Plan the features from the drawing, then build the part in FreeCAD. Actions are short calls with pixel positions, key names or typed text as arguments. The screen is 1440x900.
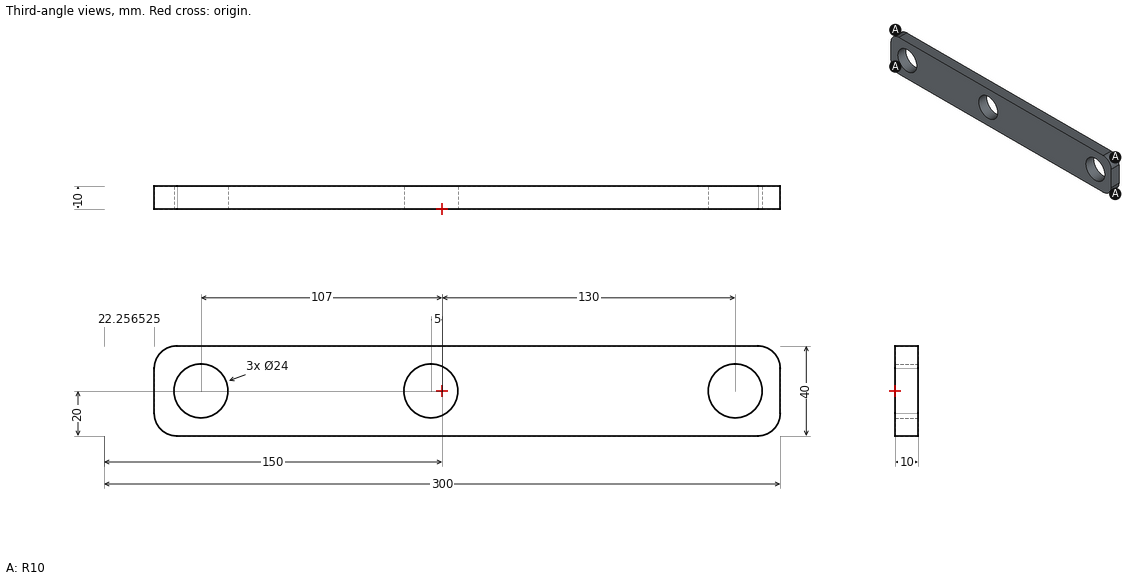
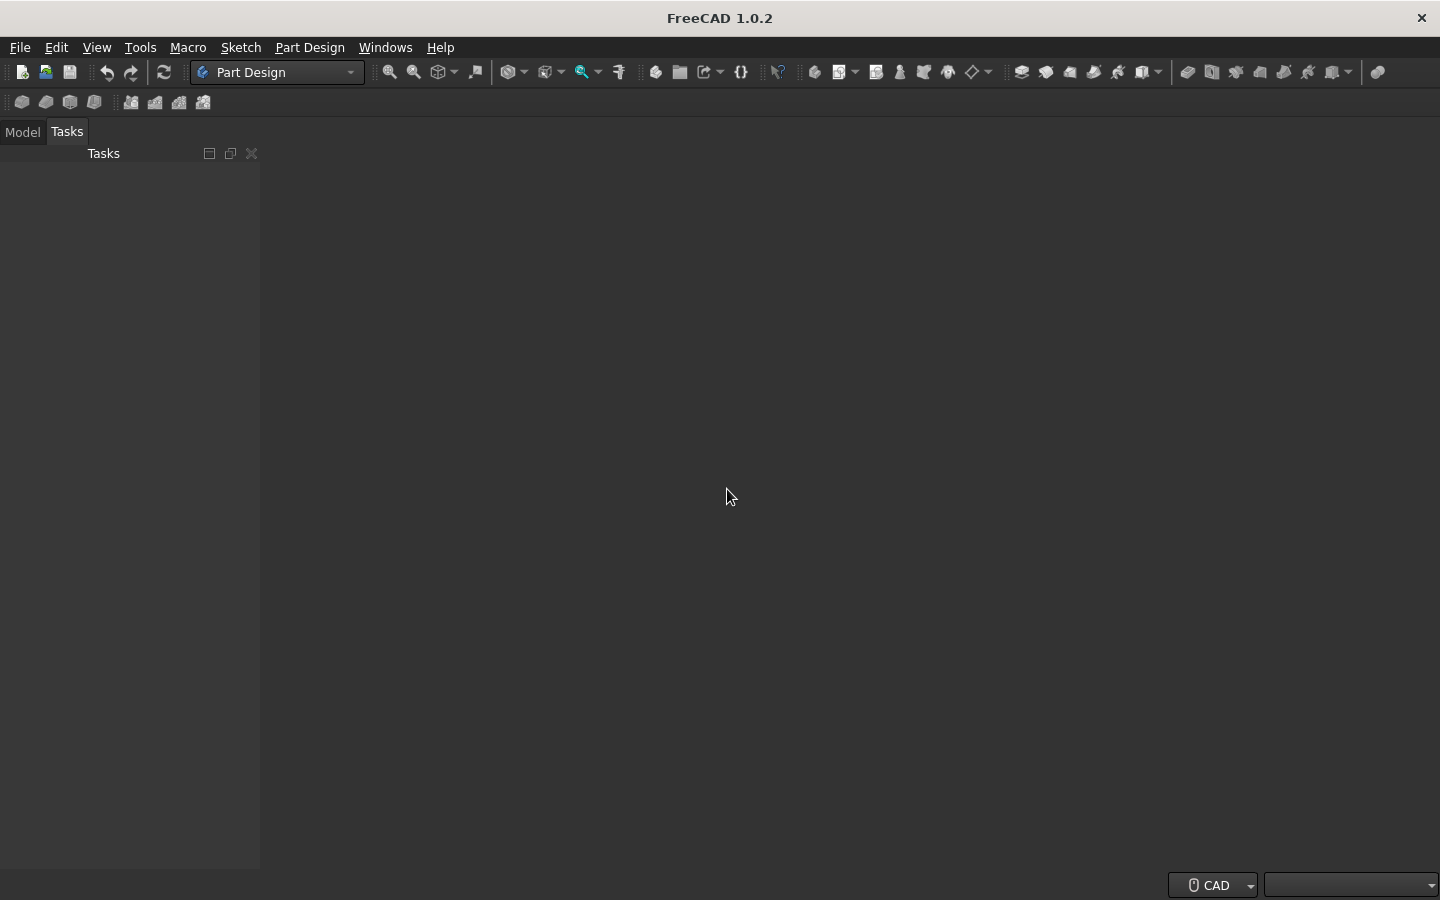
click(22, 72)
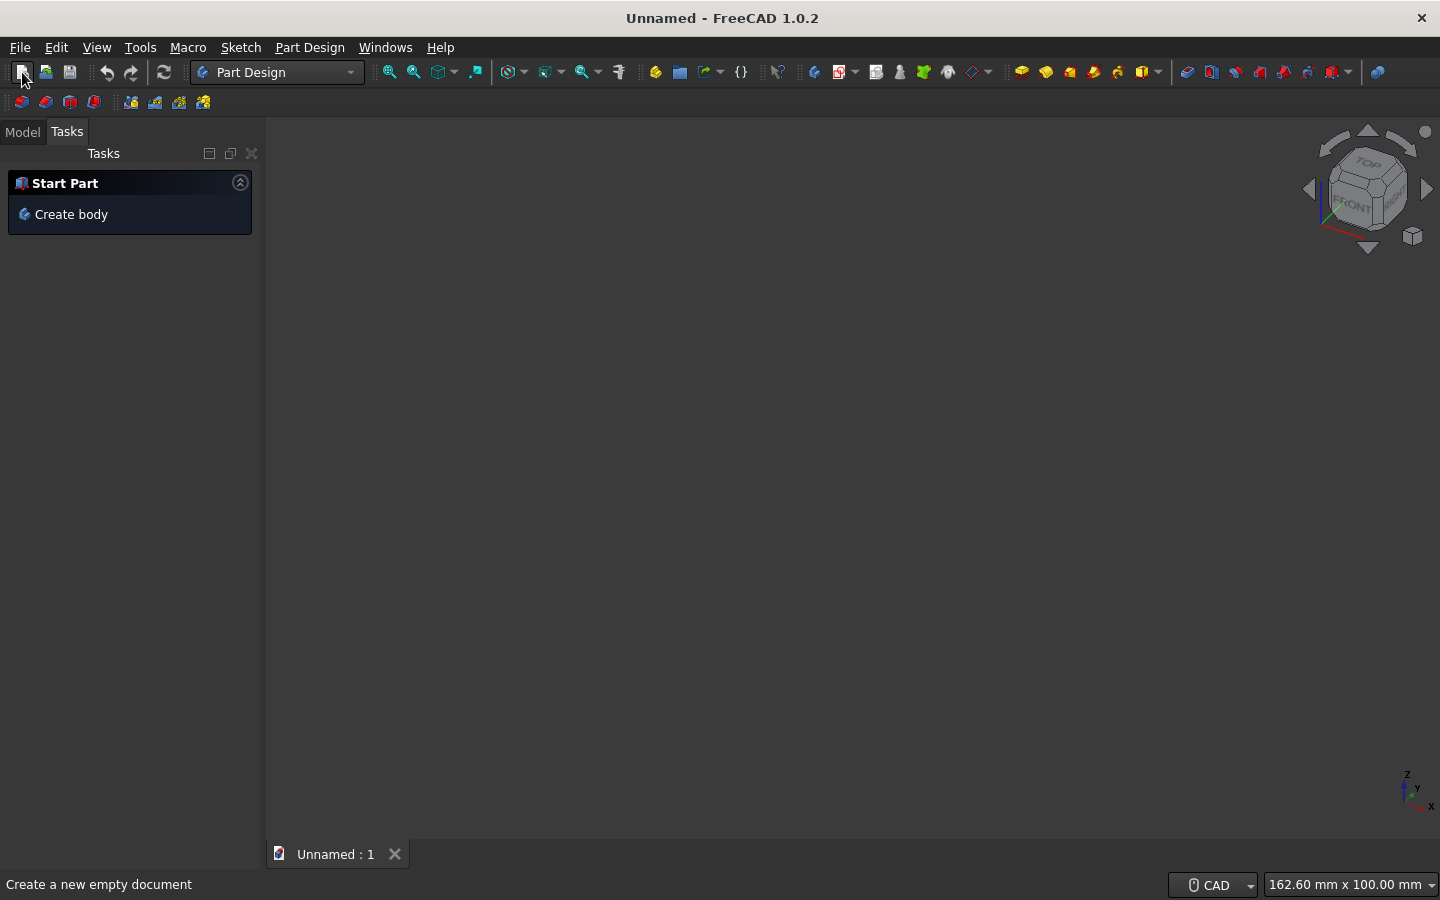
click(840, 72)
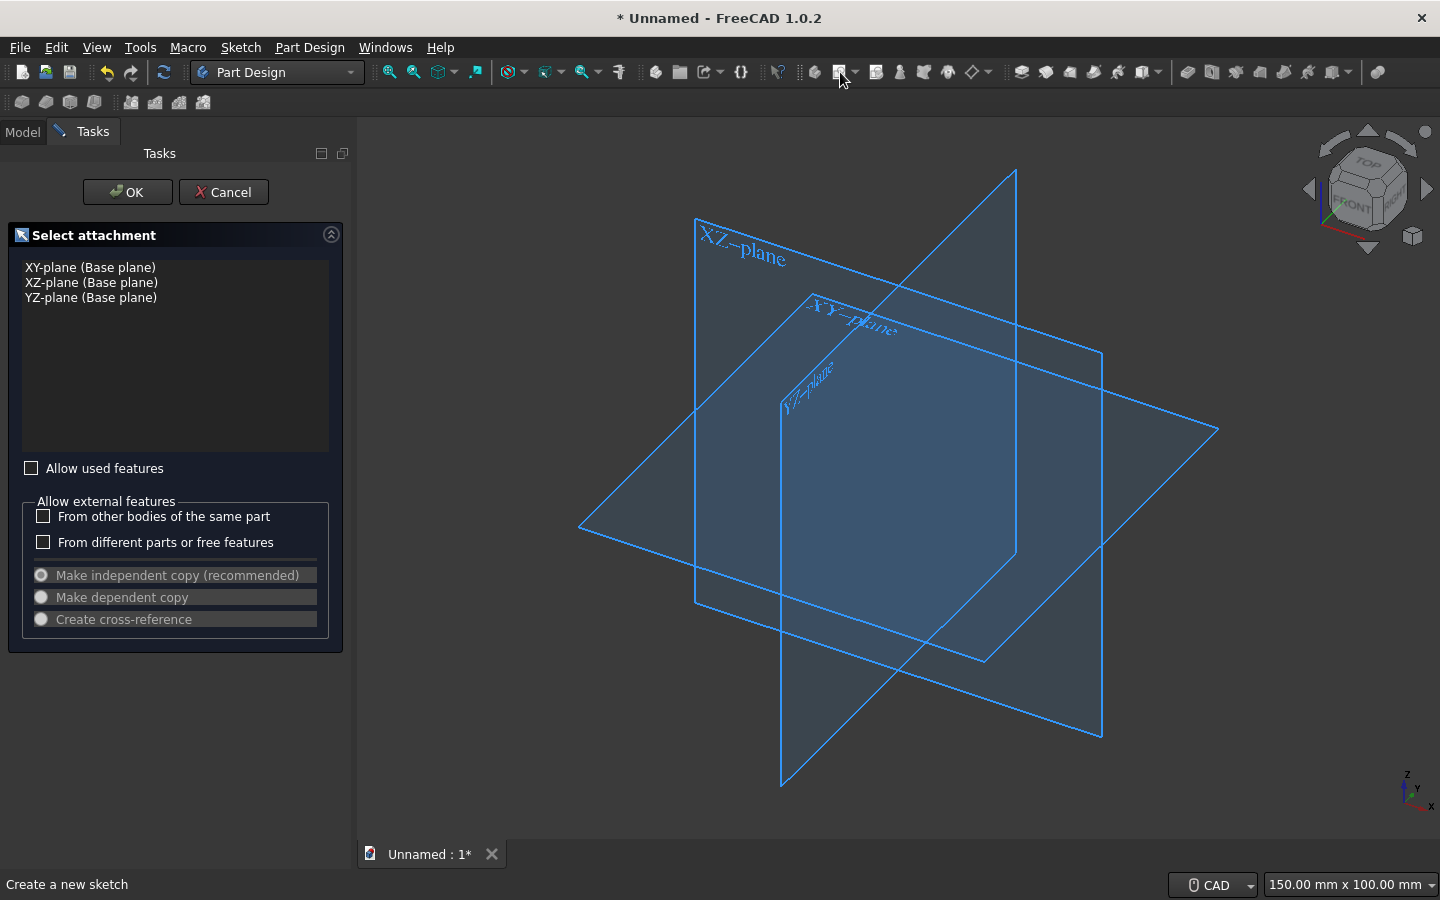
click(82, 282)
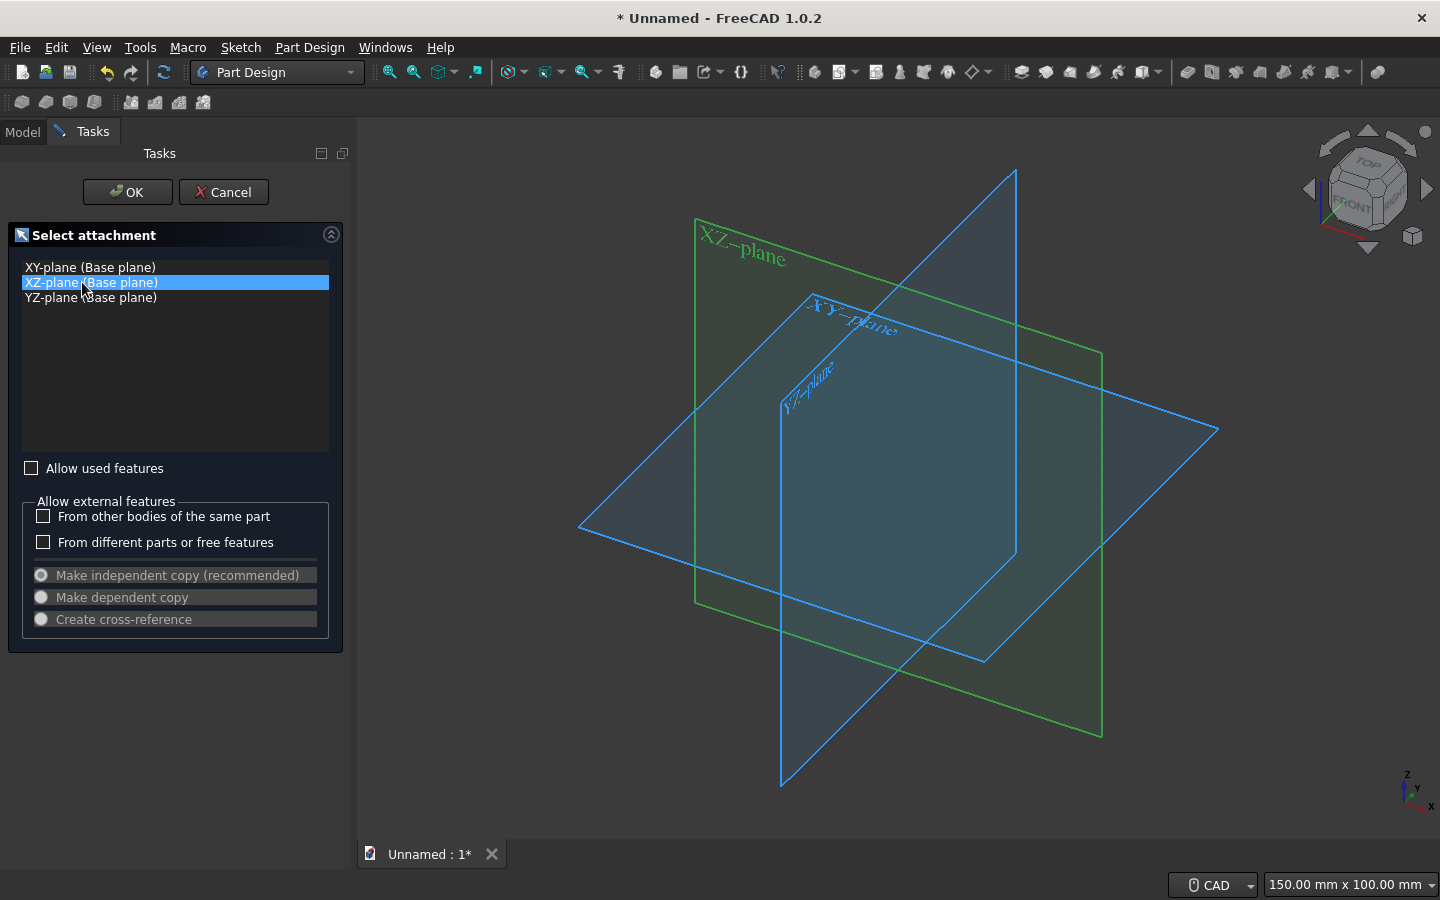
click(128, 192)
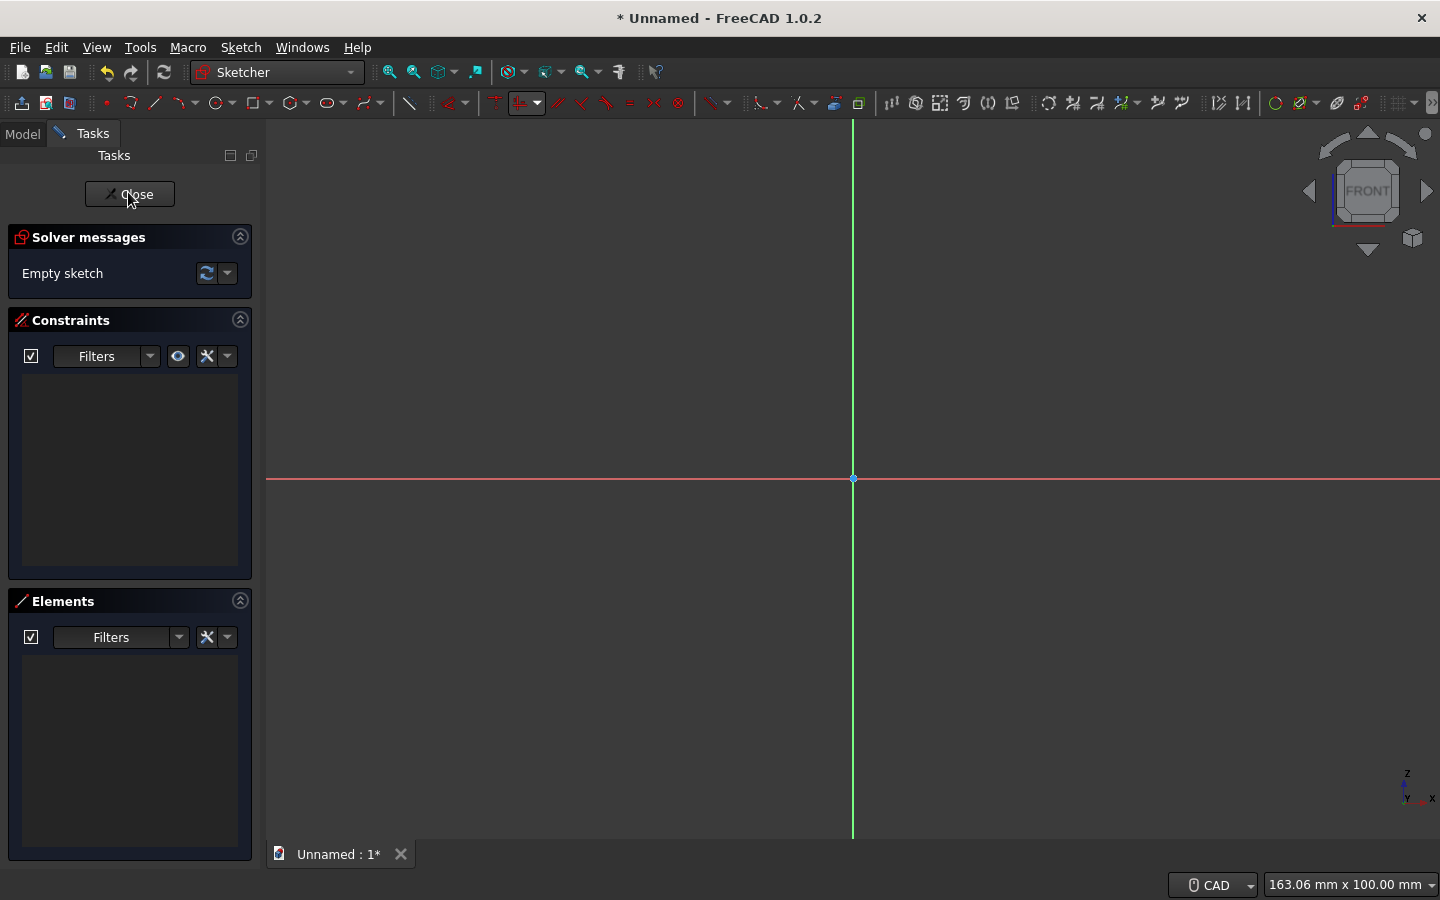
scroll(755, 479, down, 6)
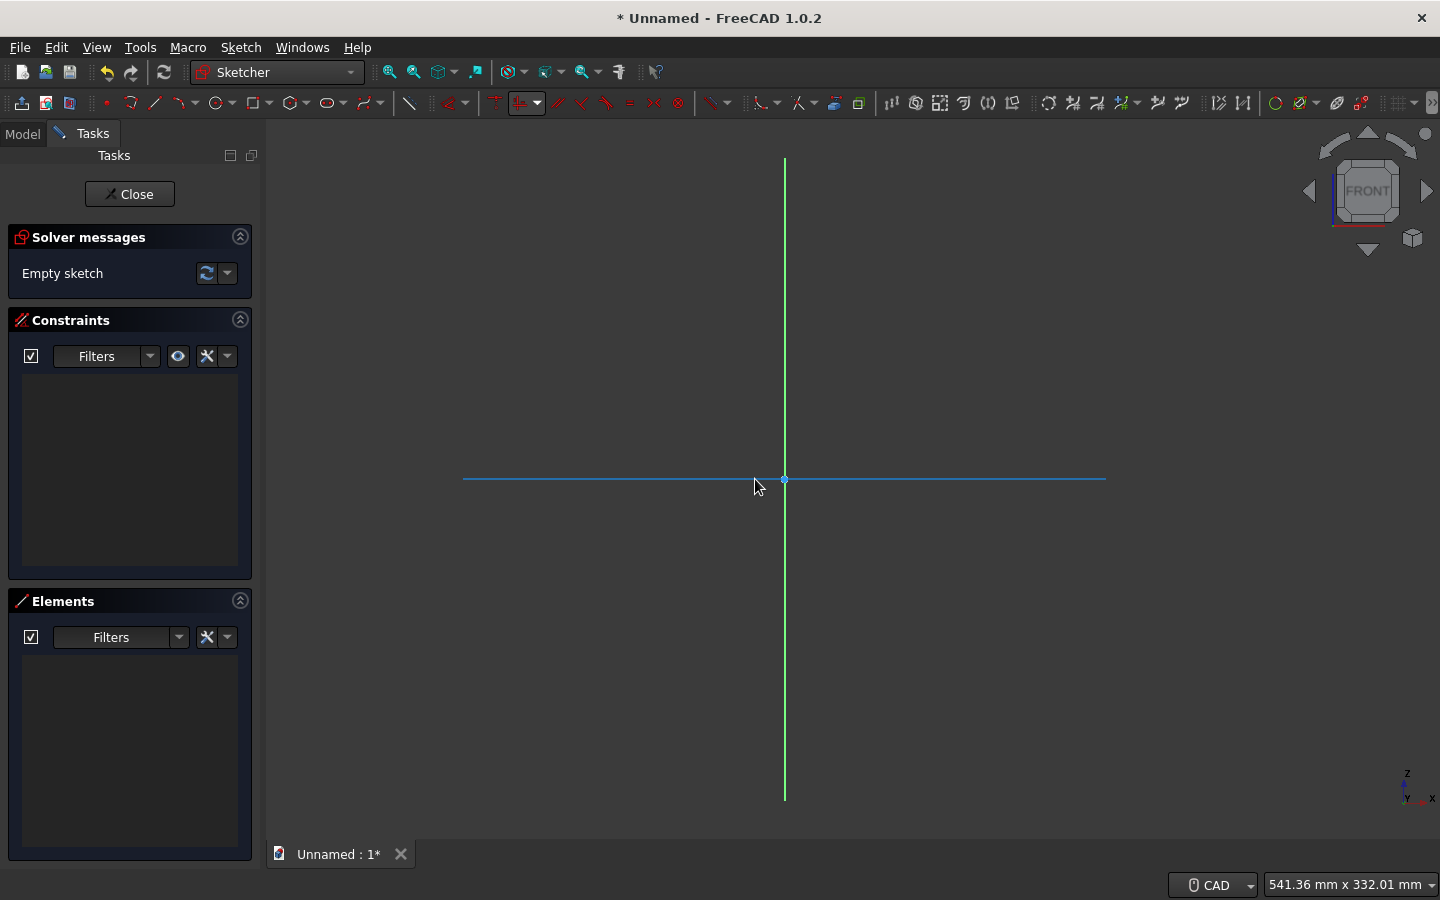
key(g)
key(v)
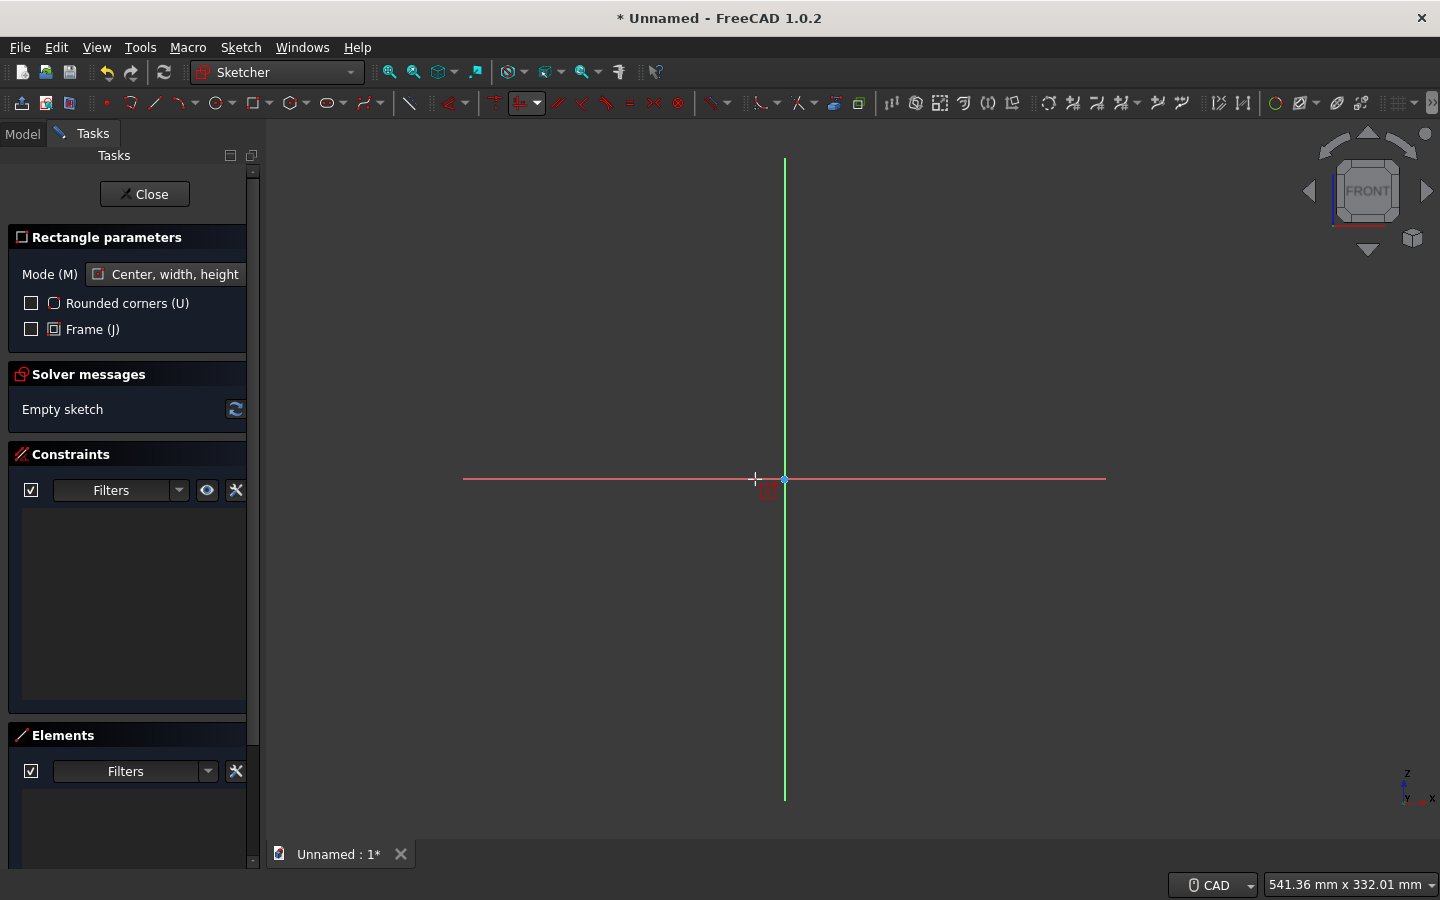
click(785, 479)
click(1110, 436)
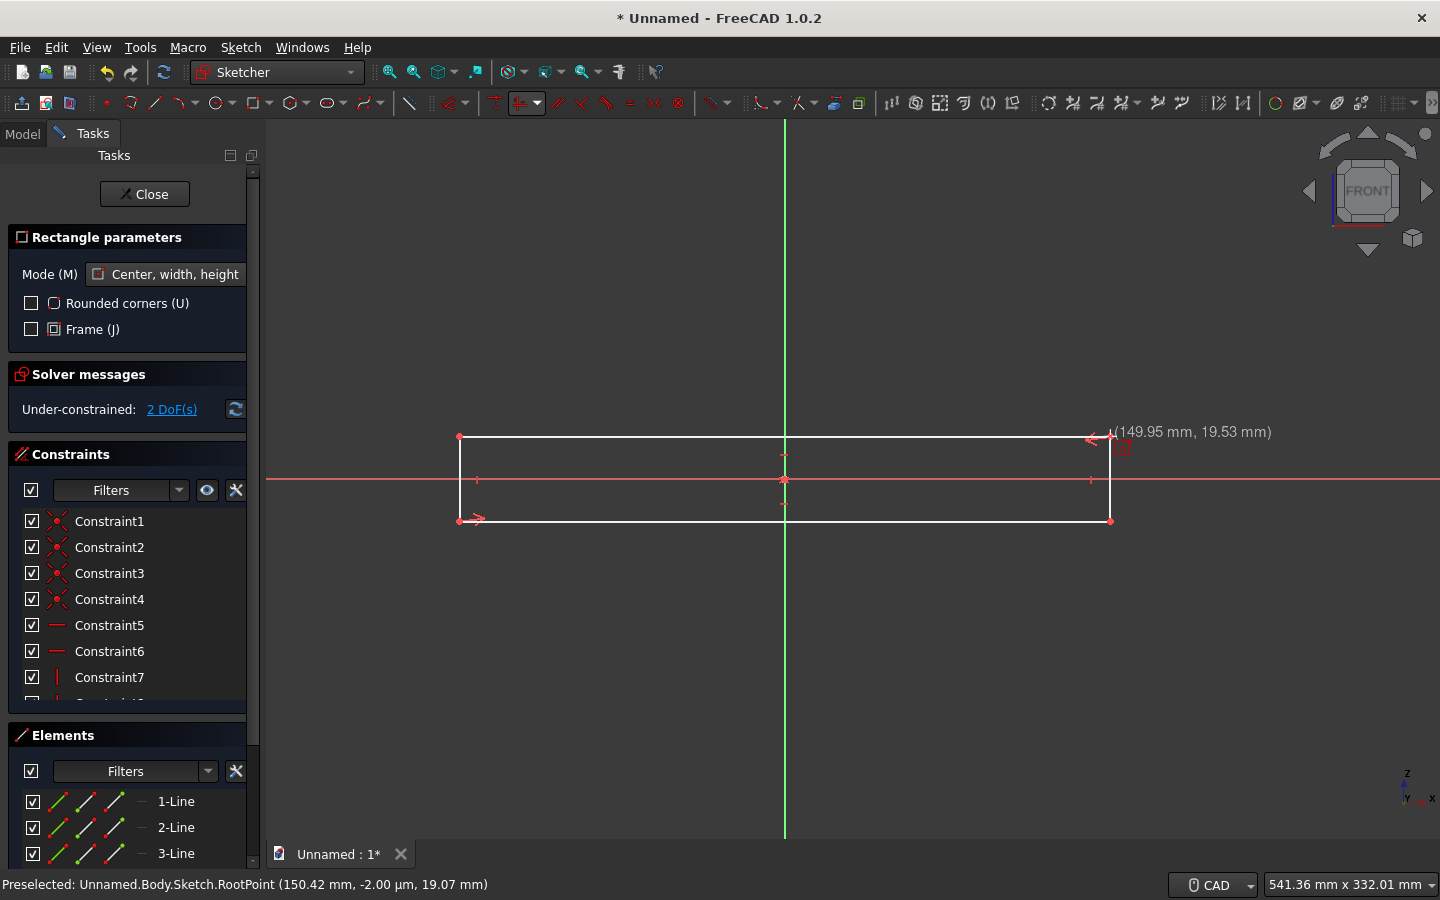
click(216, 104)